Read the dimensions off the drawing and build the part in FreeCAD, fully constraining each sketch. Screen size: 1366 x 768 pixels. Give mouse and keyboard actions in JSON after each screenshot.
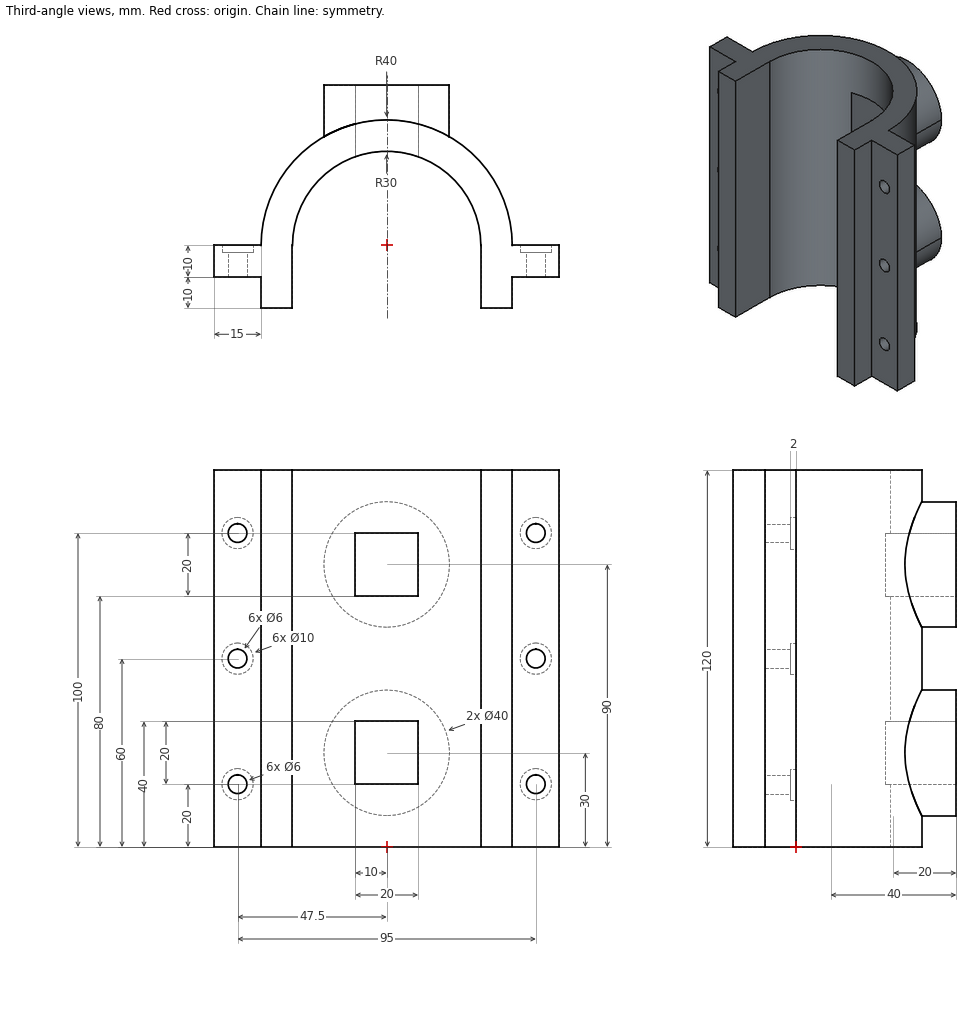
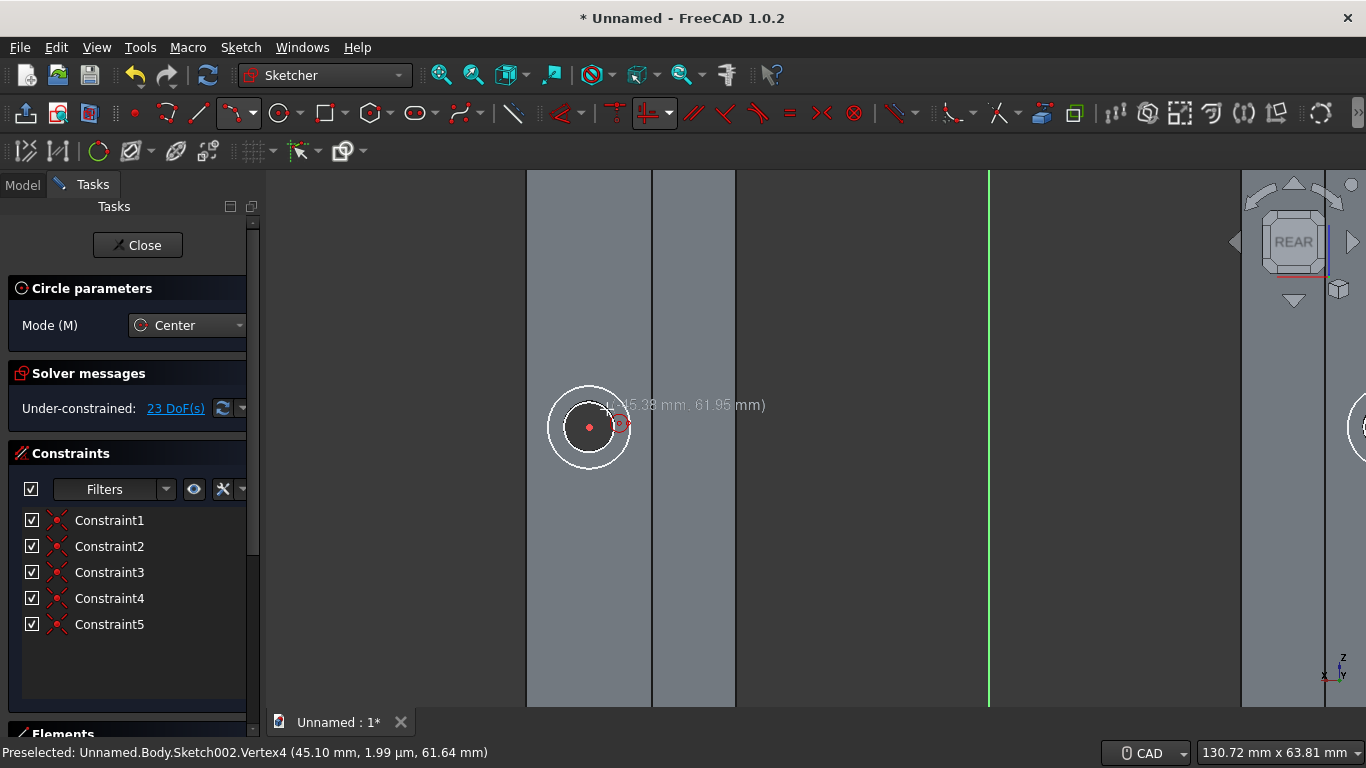
{"action": "scroll", "coordinate": [607, 409], "scroll_direction": "down", "scroll_amount": 5}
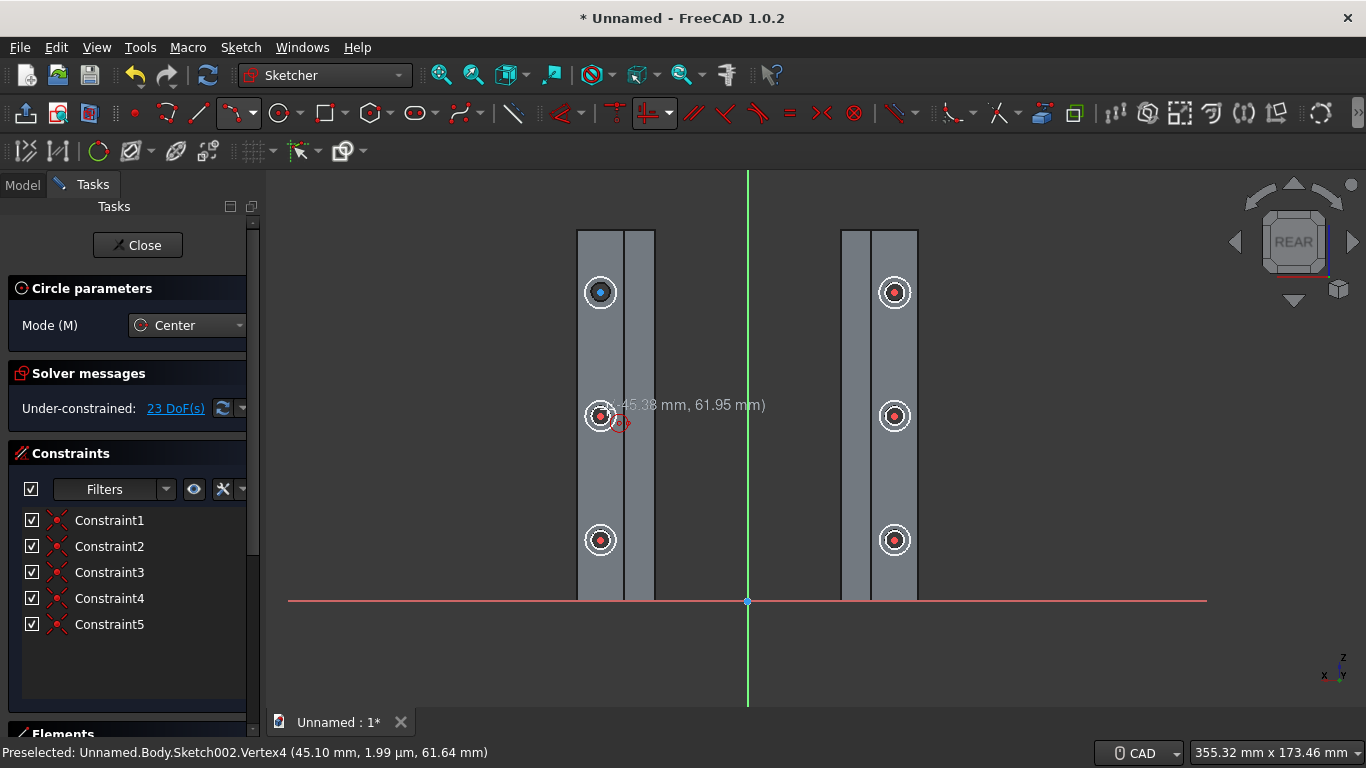
{"action": "scroll", "coordinate": [601, 292], "scroll_direction": "up", "scroll_amount": 5}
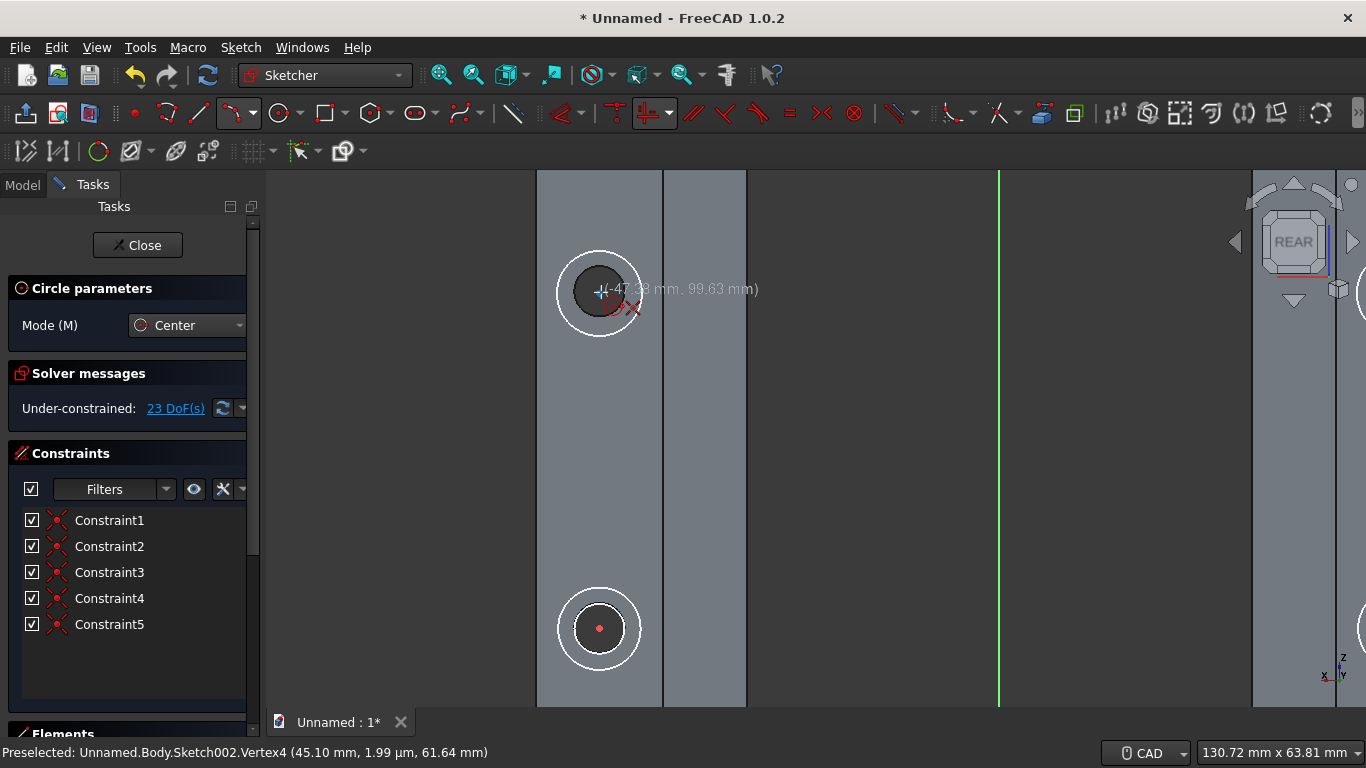
{"action": "left_click", "coordinate": [599, 294]}
{"action": "left_click", "coordinate": [617, 273]}
{"action": "key", "text": "Escape"}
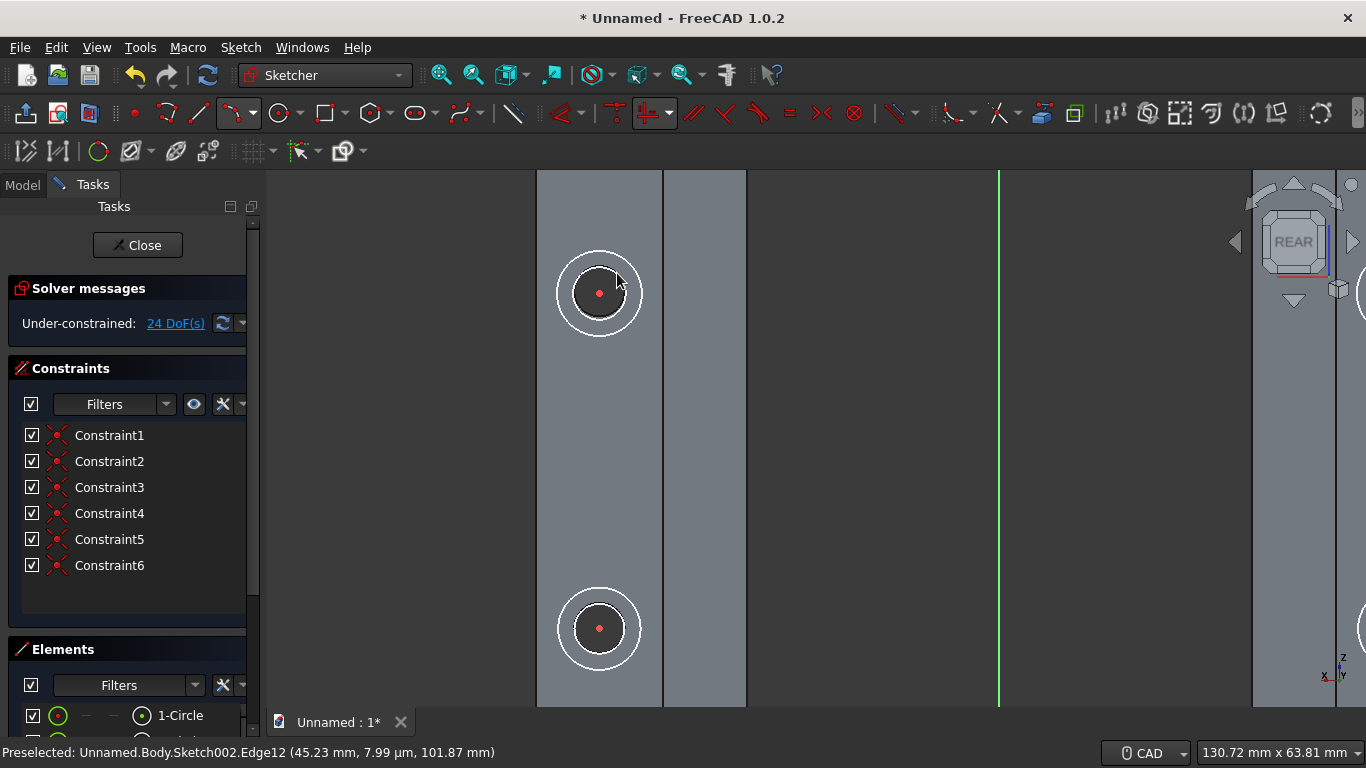
{"action": "scroll", "coordinate": [601, 292], "scroll_direction": "down", "scroll_amount": 5}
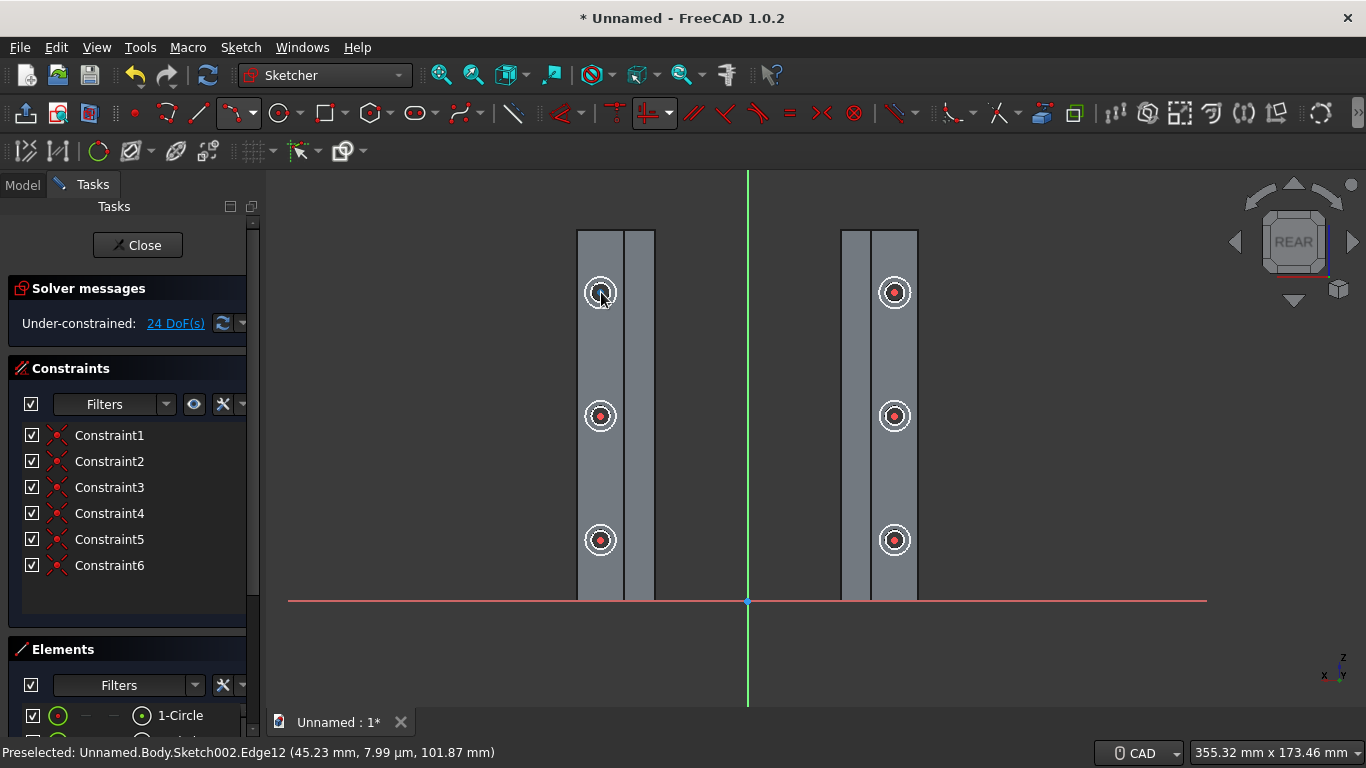
{"action": "scroll", "coordinate": [906, 405], "scroll_direction": "up", "scroll_amount": 5}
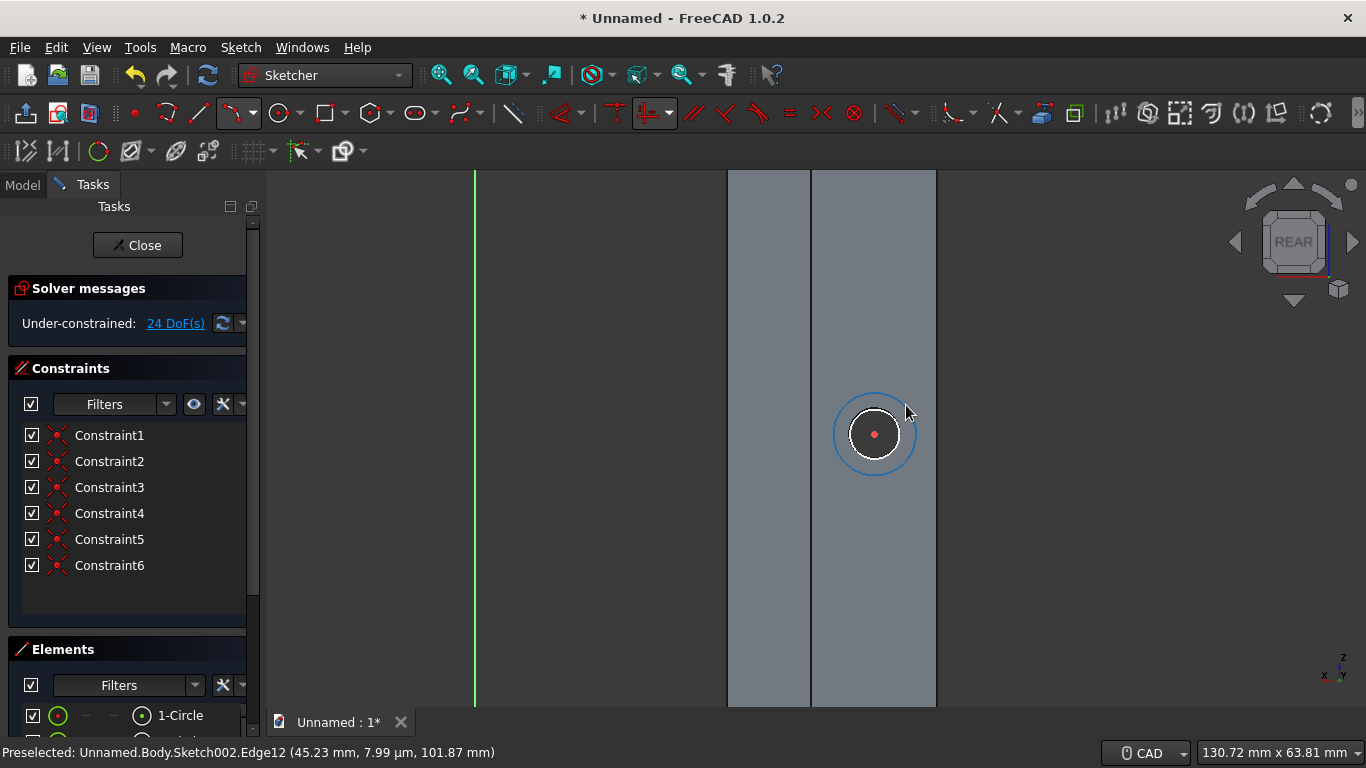
{"action": "left_click", "coordinate": [904, 405]}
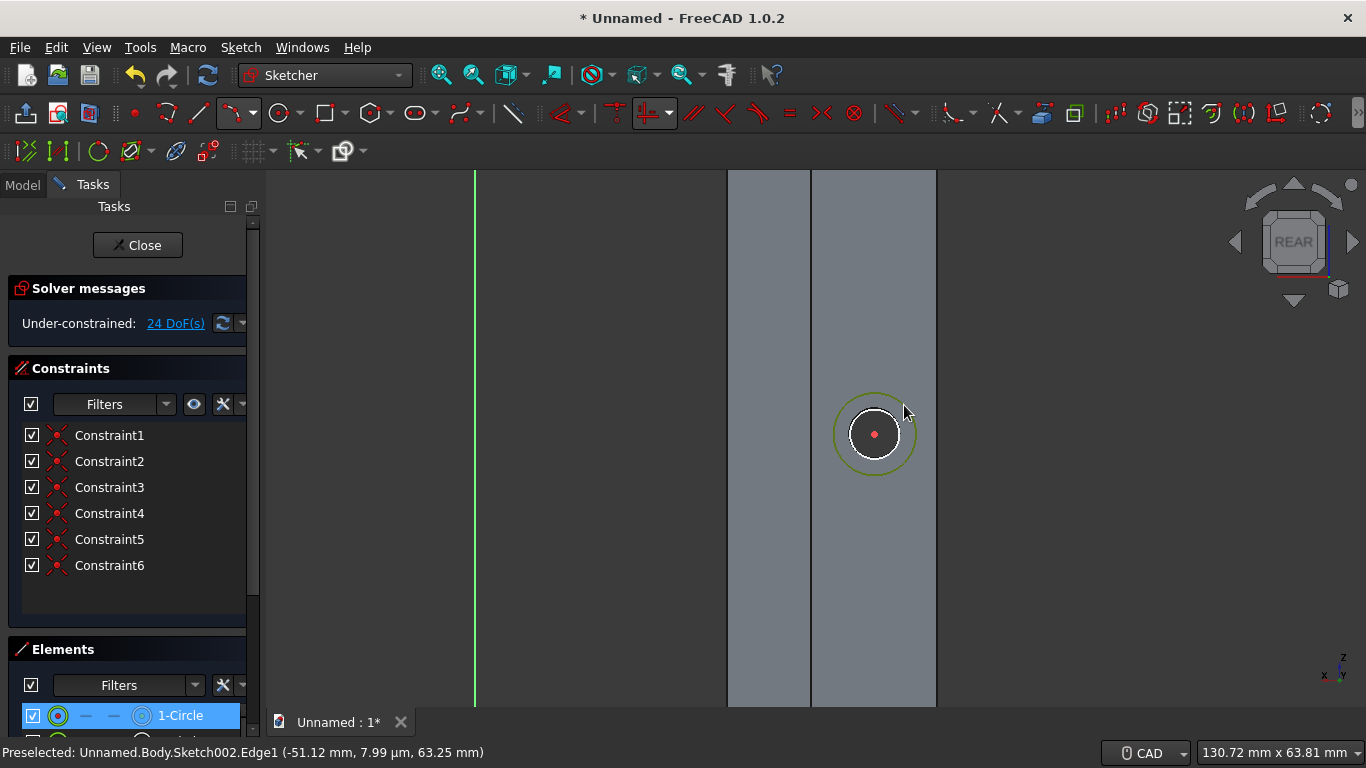
{"action": "scroll", "coordinate": [906, 405], "scroll_direction": "down", "scroll_amount": 5}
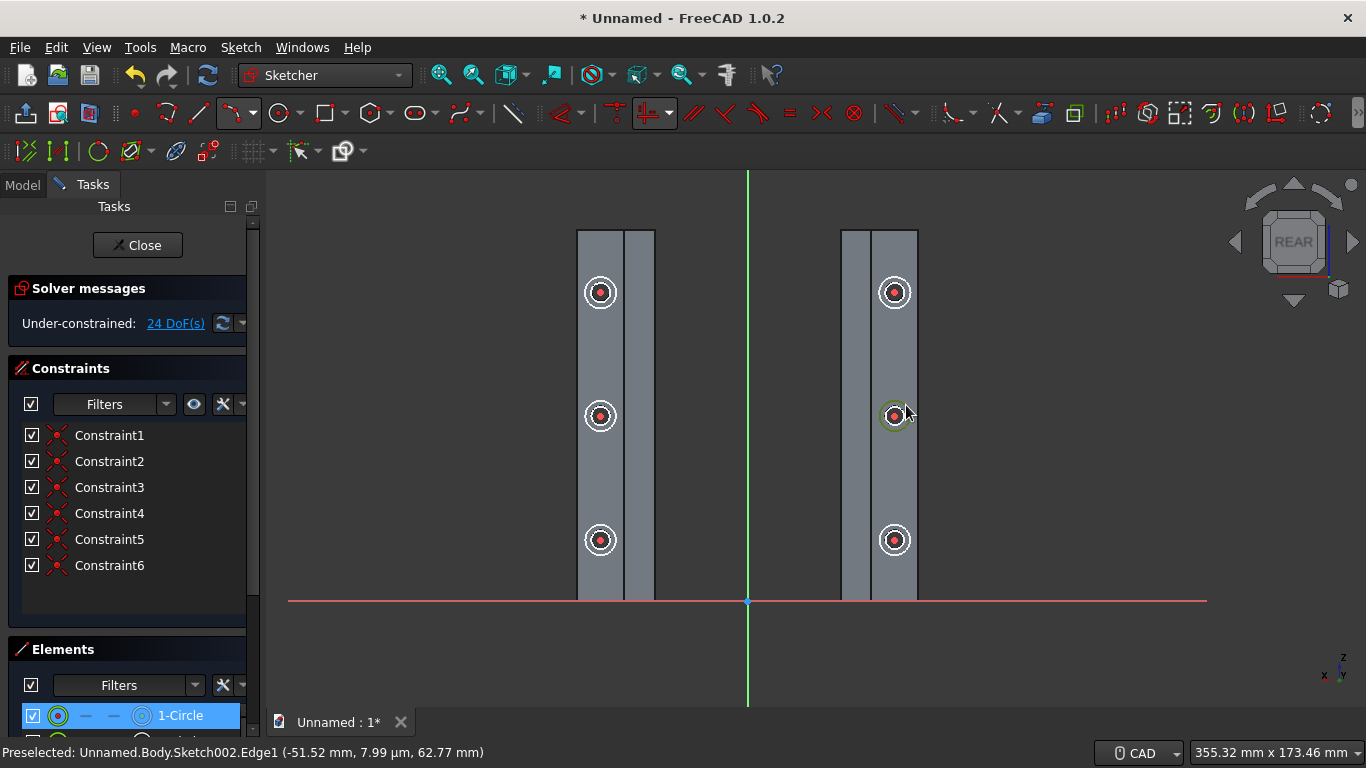
{"action": "scroll", "coordinate": [906, 282], "scroll_direction": "up", "scroll_amount": 5}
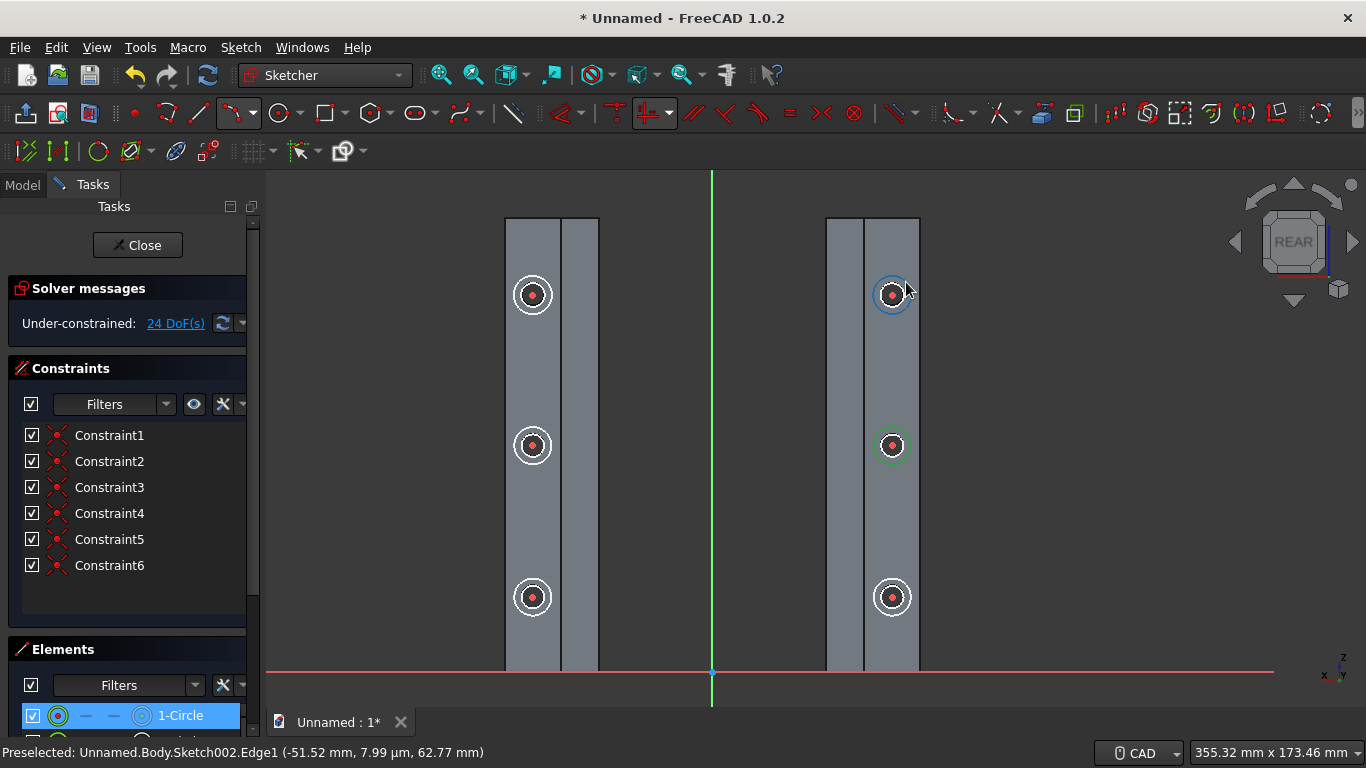
{"action": "left_click", "coordinate": [905, 281]}